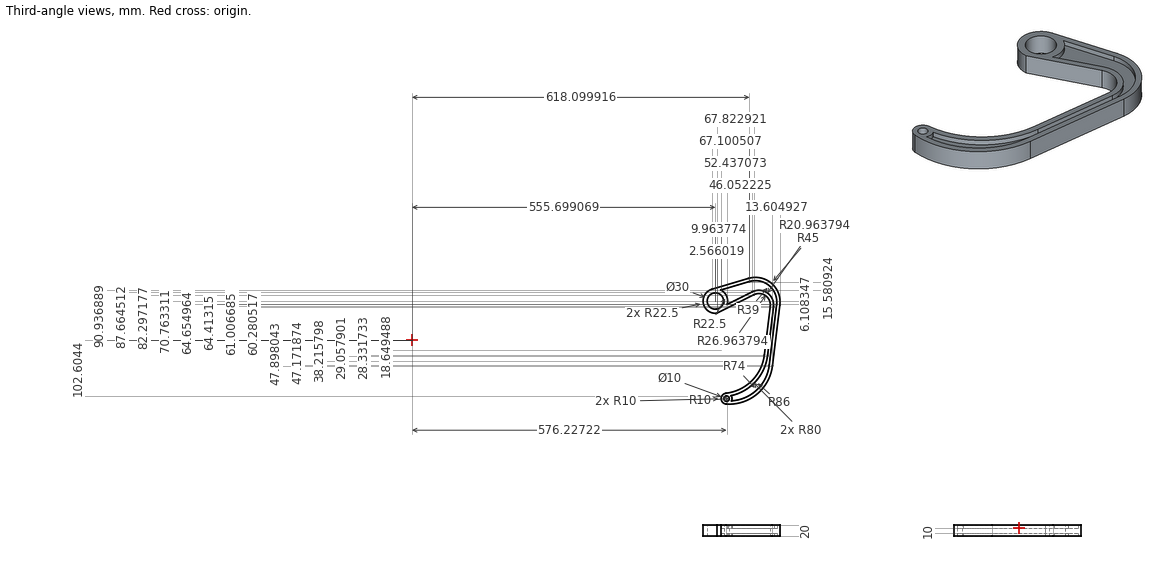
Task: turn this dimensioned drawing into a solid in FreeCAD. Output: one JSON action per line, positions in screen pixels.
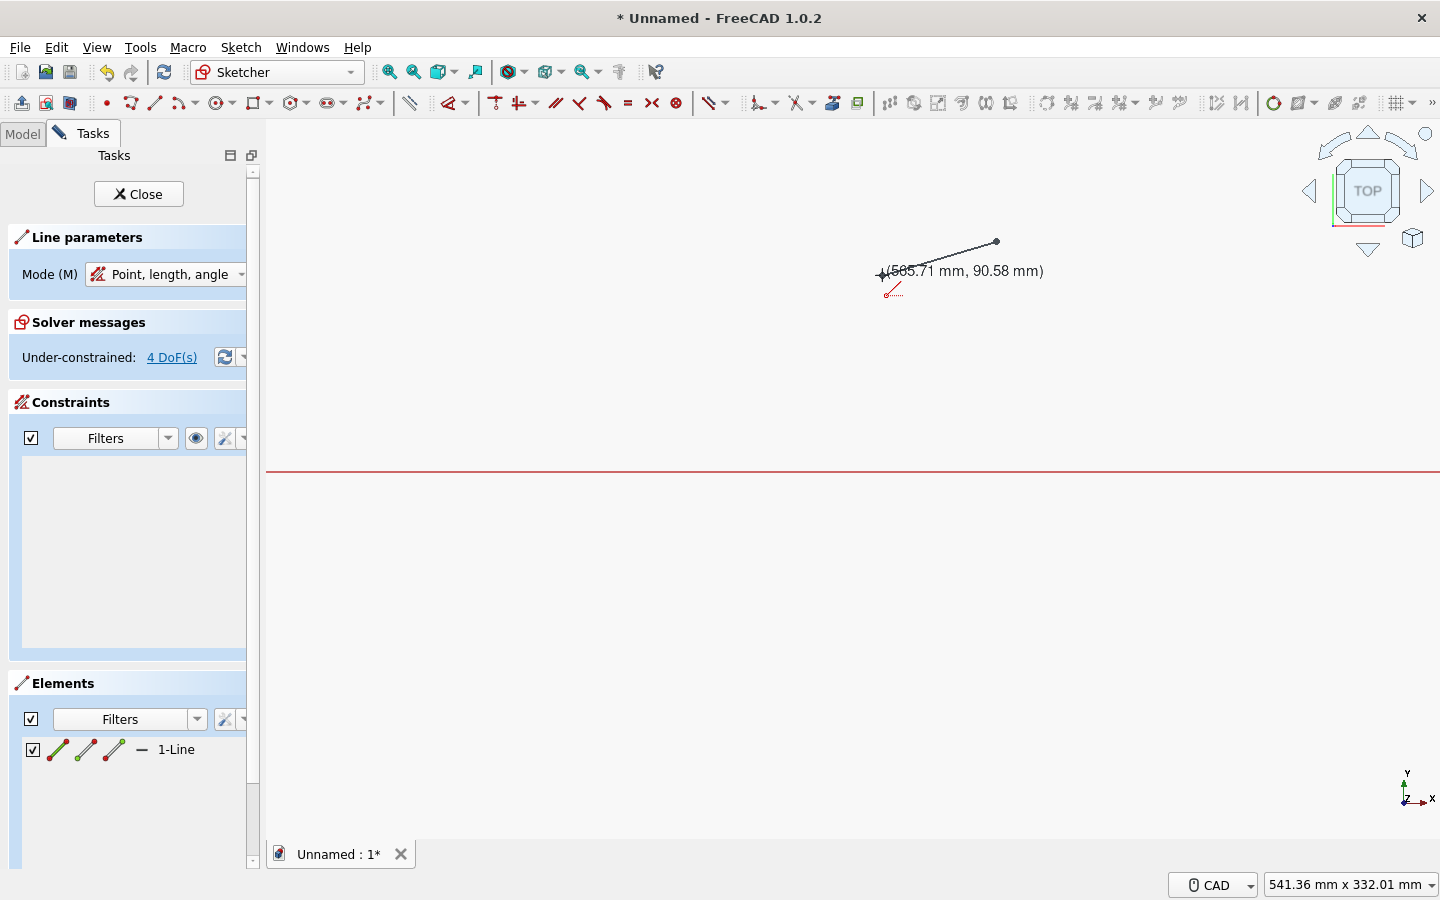
{"action": "left_click", "coordinate": [907, 332]}
{"action": "left_click", "coordinate": [1007, 282]}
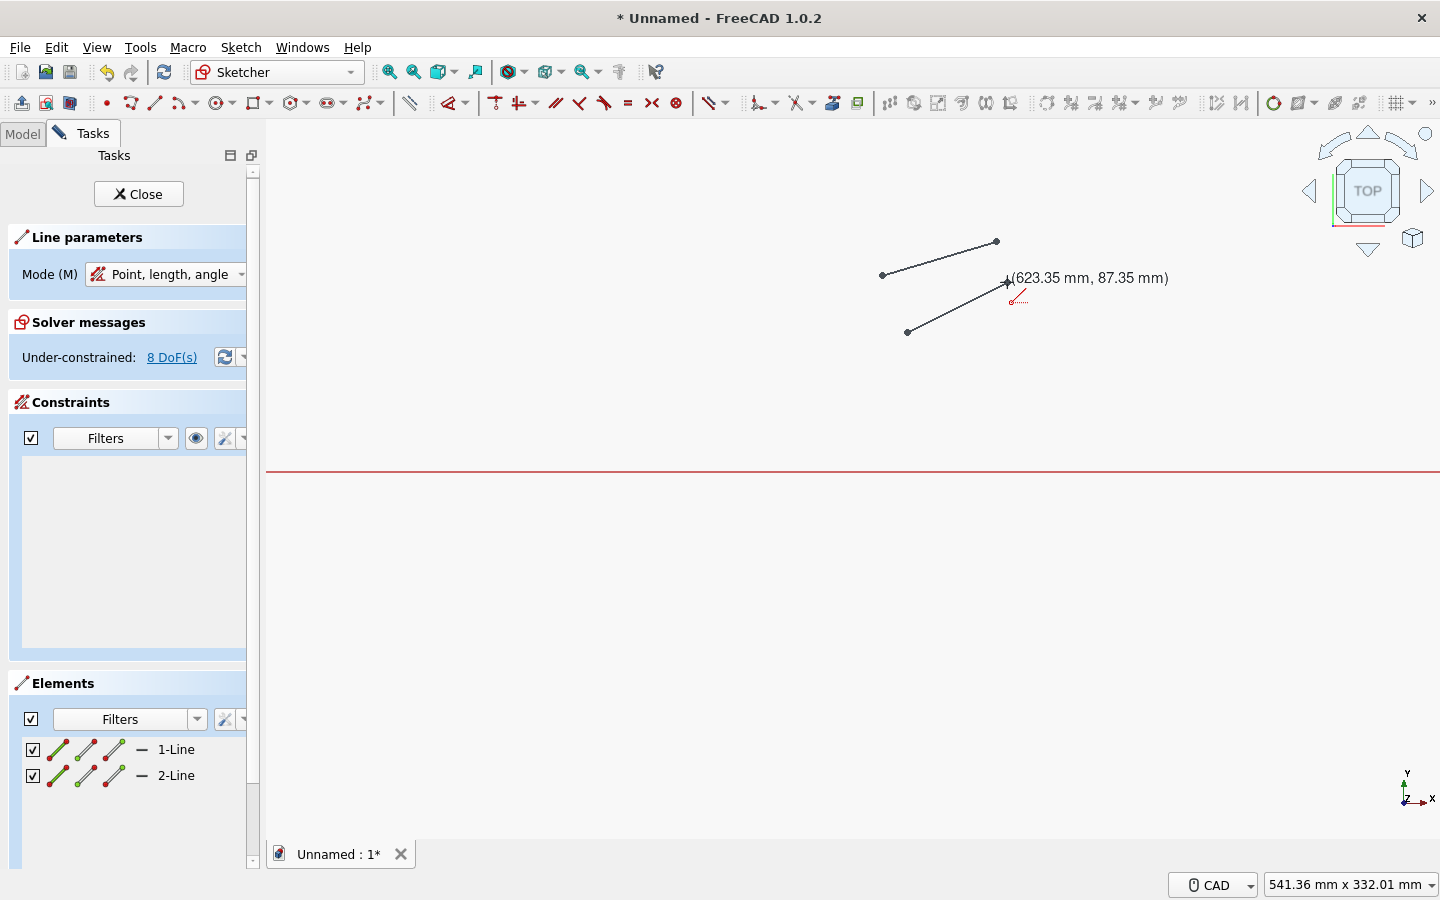
{"action": "left_click", "coordinate": [1091, 342]}
{"action": "left_click", "coordinate": [1068, 535]}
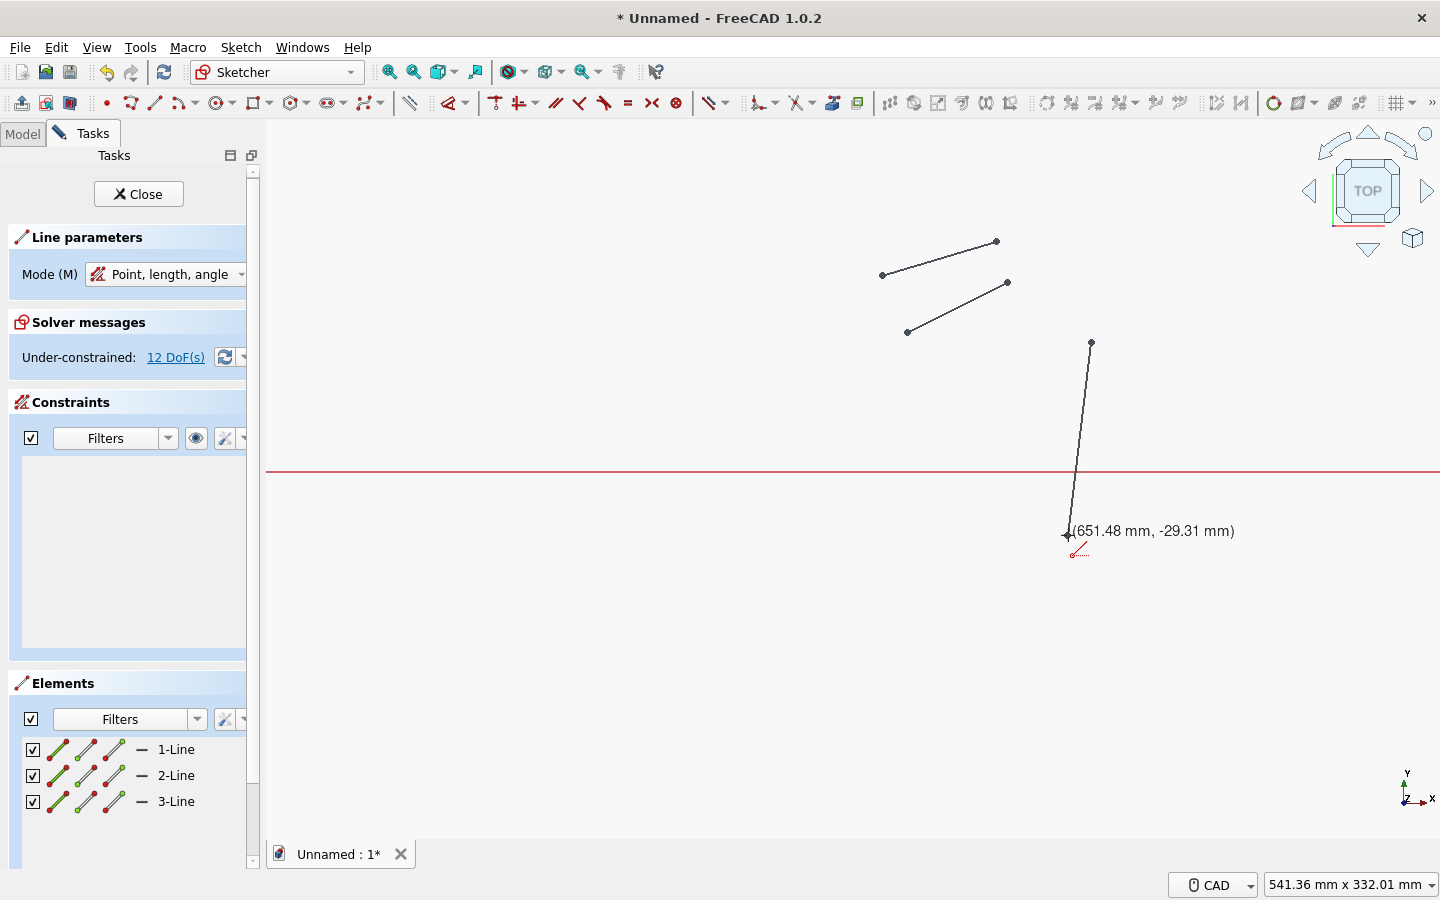
{"action": "left_click", "coordinate": [1074, 575]}
{"action": "left_click", "coordinate": [1104, 333]}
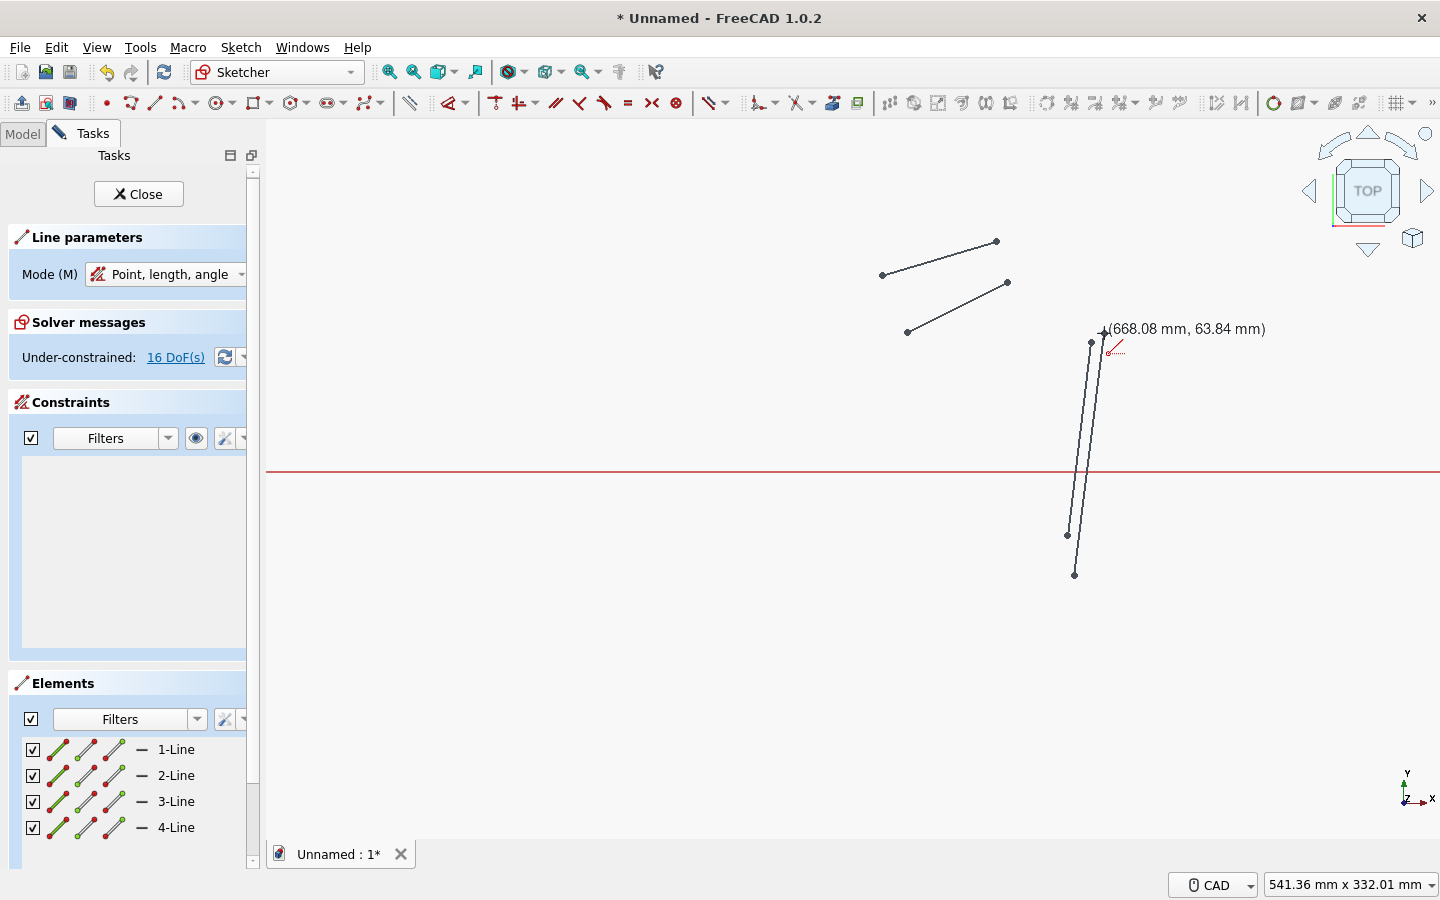
{"action": "key", "text": "g 3 a"}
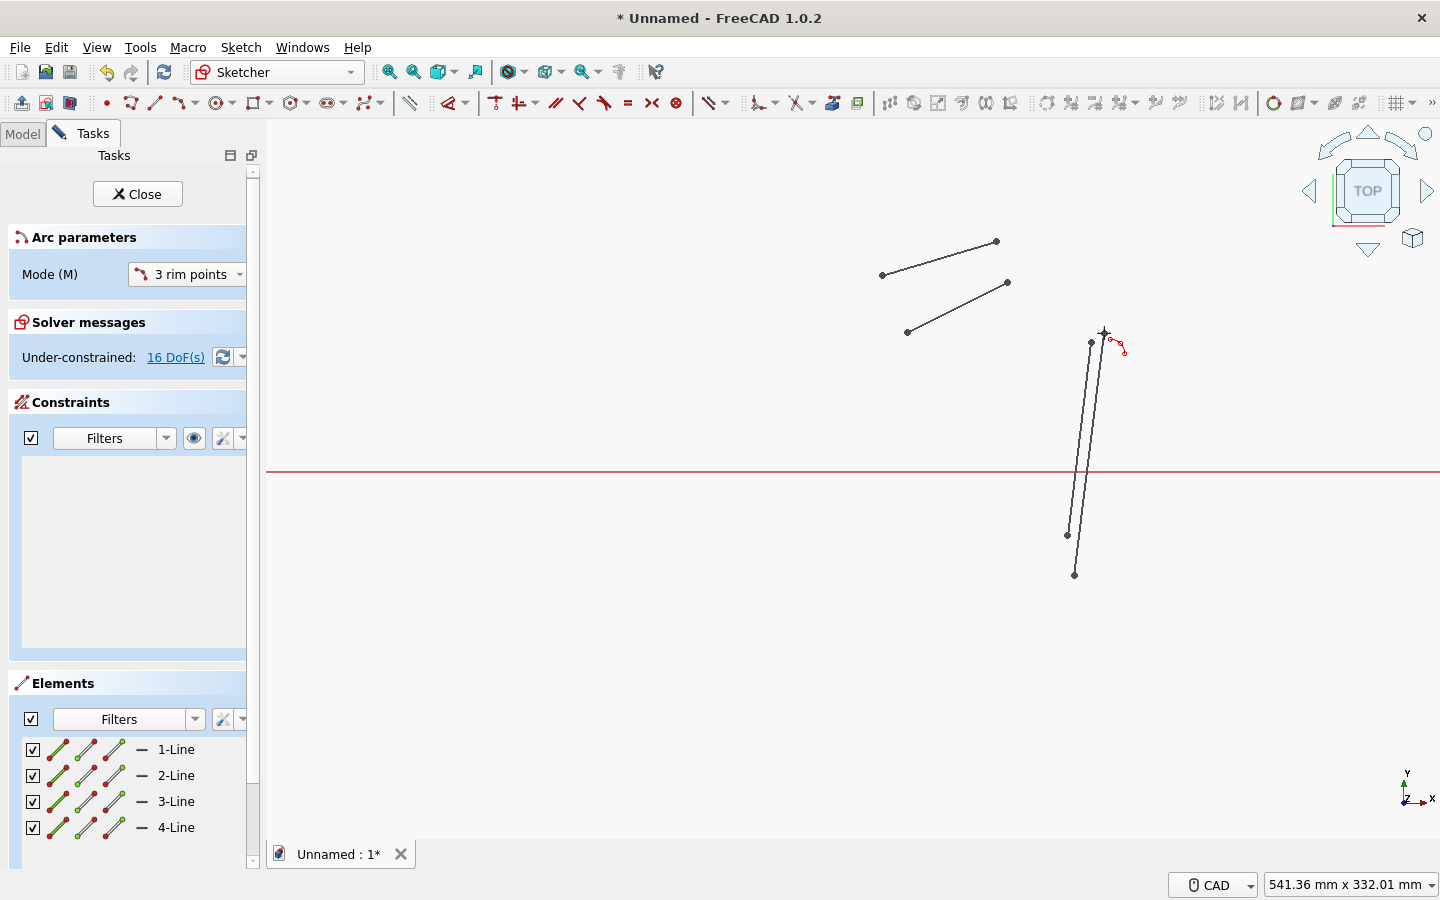
{"action": "left_click", "coordinate": [882, 276]}
{"action": "left_click", "coordinate": [907, 333]}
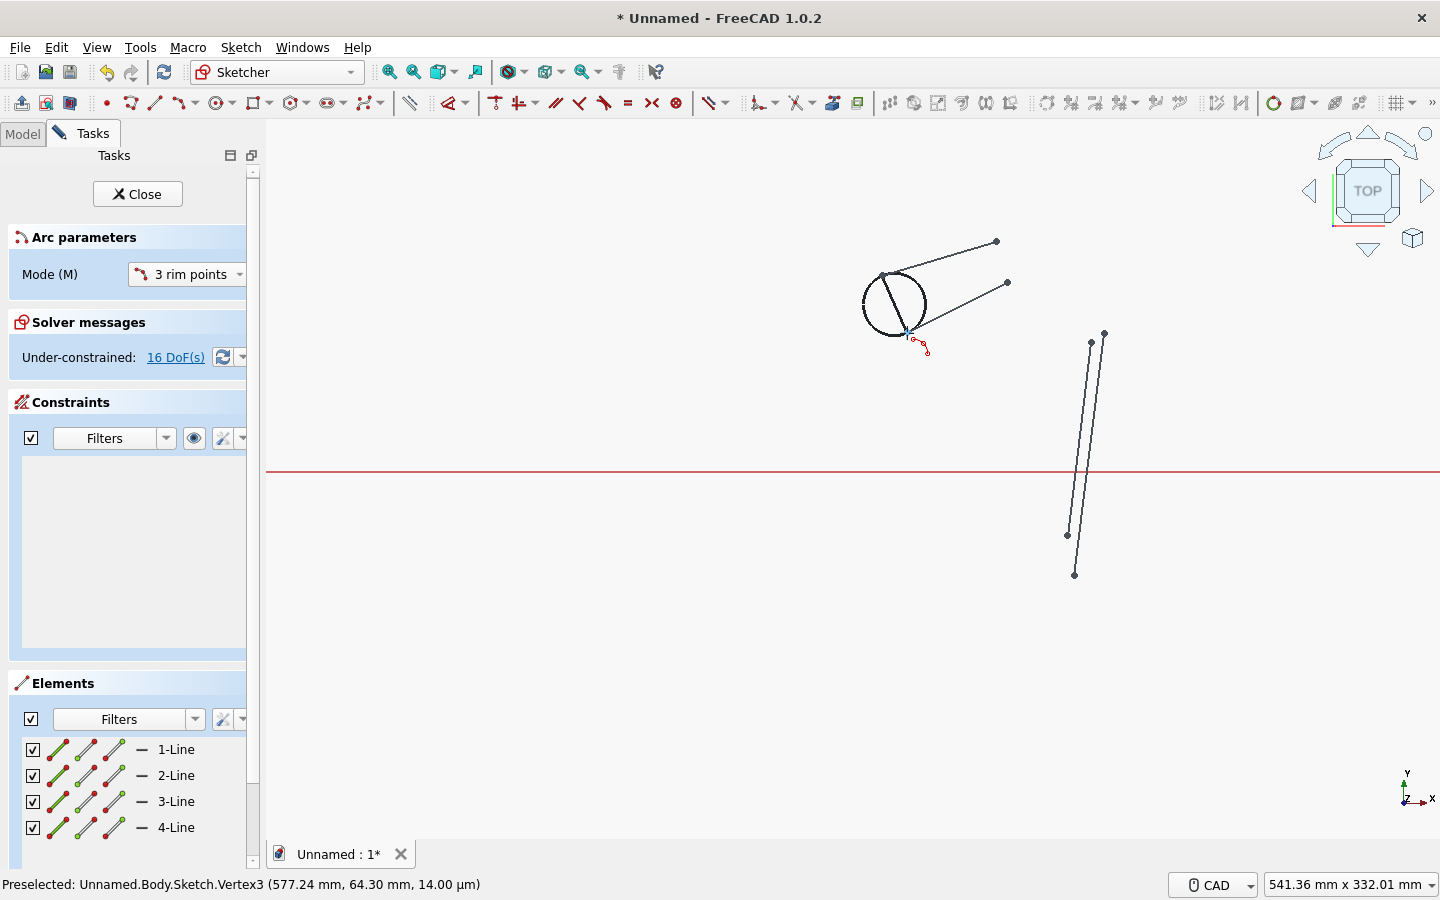
{"action": "scroll", "coordinate": [905, 299], "scroll_direction": "up", "scroll_amount": 2}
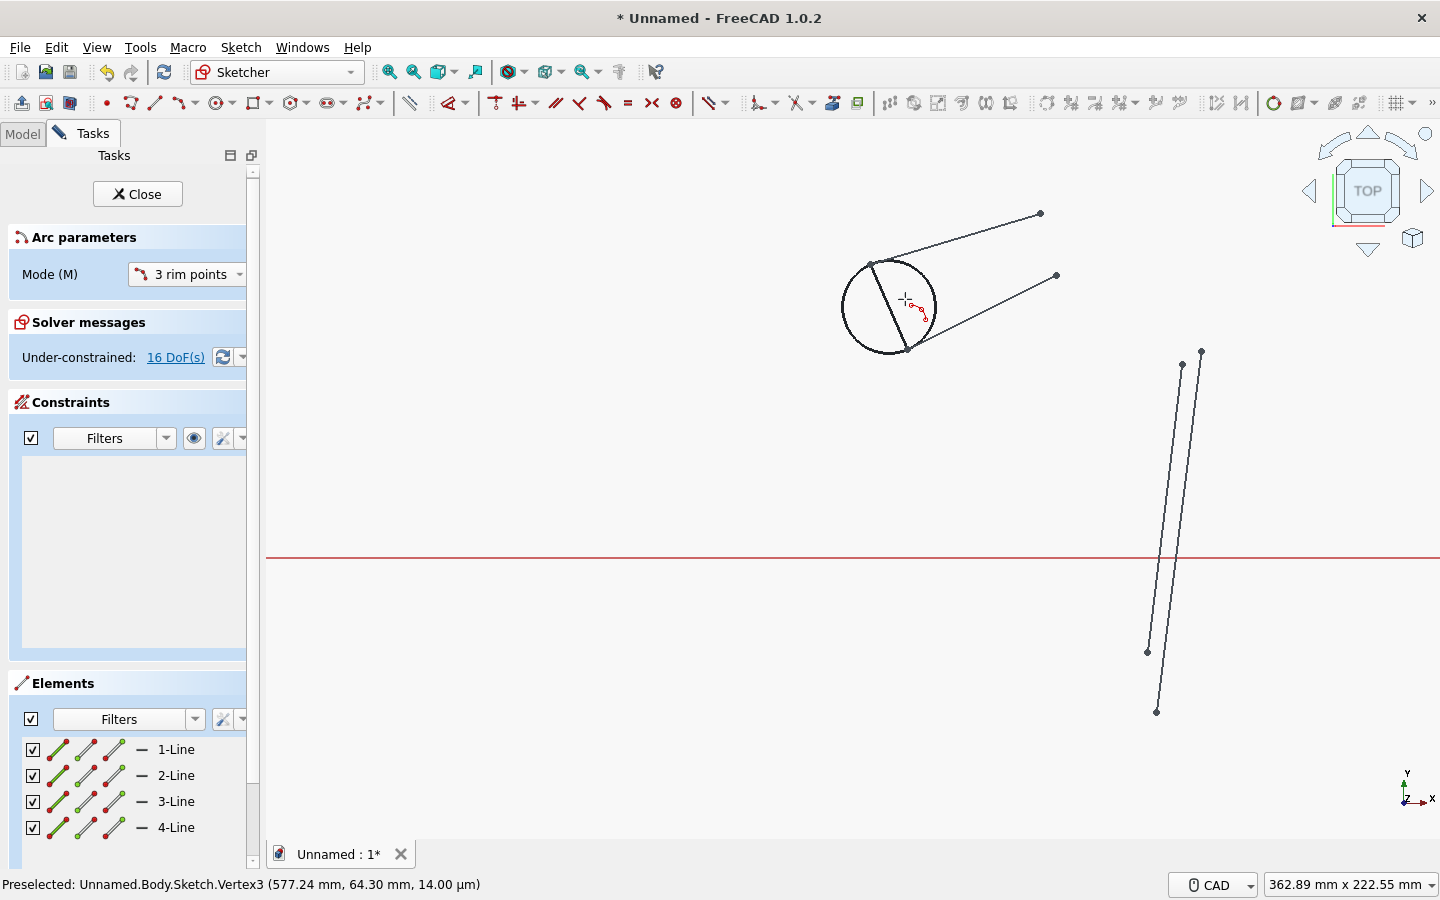
{"action": "left_click", "coordinate": [905, 299]}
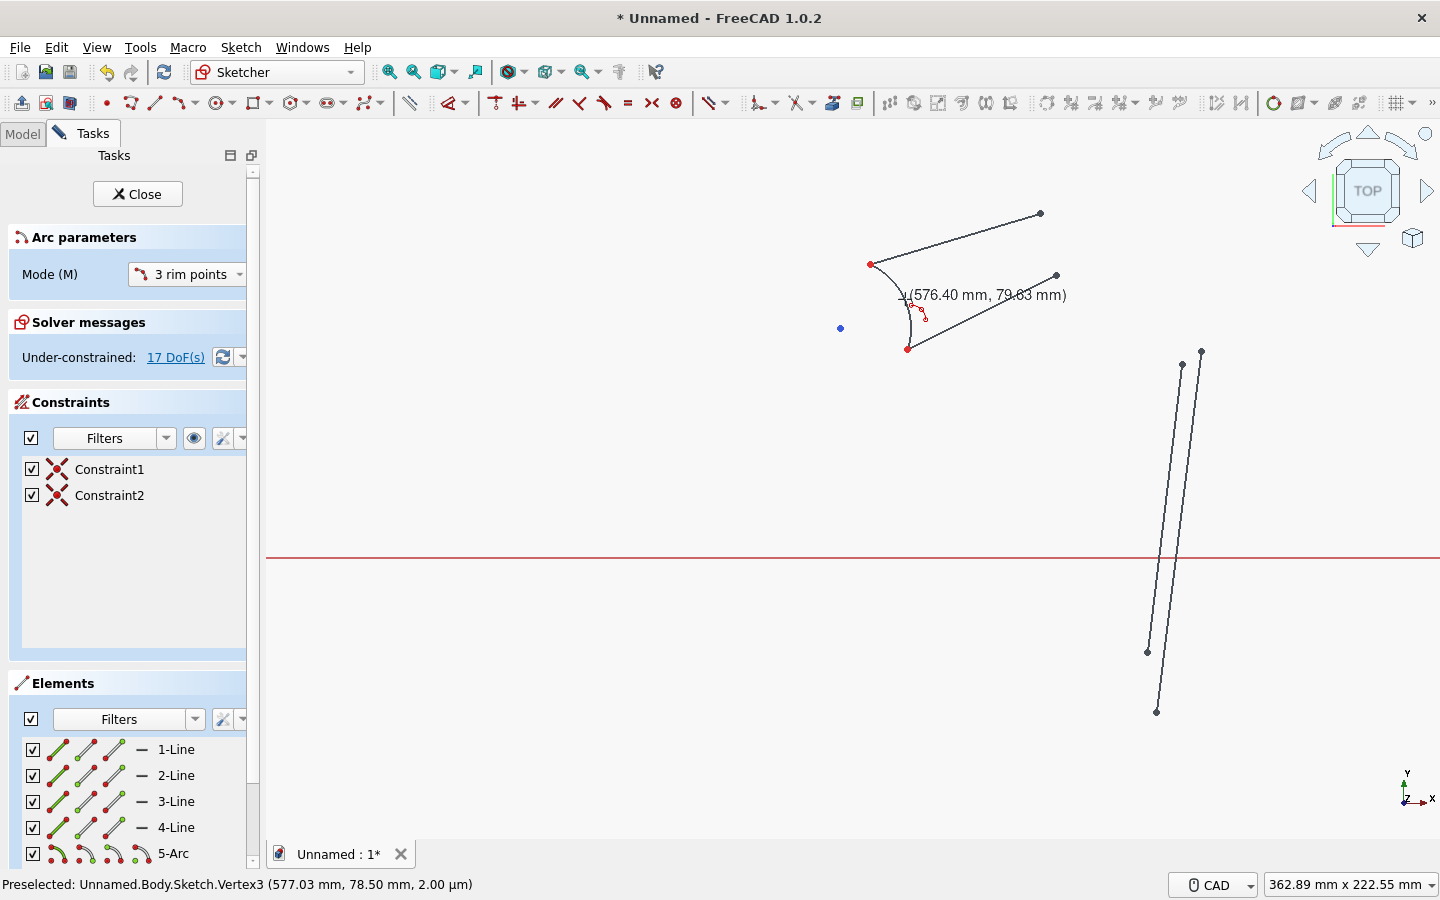
{"action": "left_click", "coordinate": [1057, 275]}
{"action": "left_click", "coordinate": [1182, 365]}
{"action": "left_click", "coordinate": [1146, 281]}